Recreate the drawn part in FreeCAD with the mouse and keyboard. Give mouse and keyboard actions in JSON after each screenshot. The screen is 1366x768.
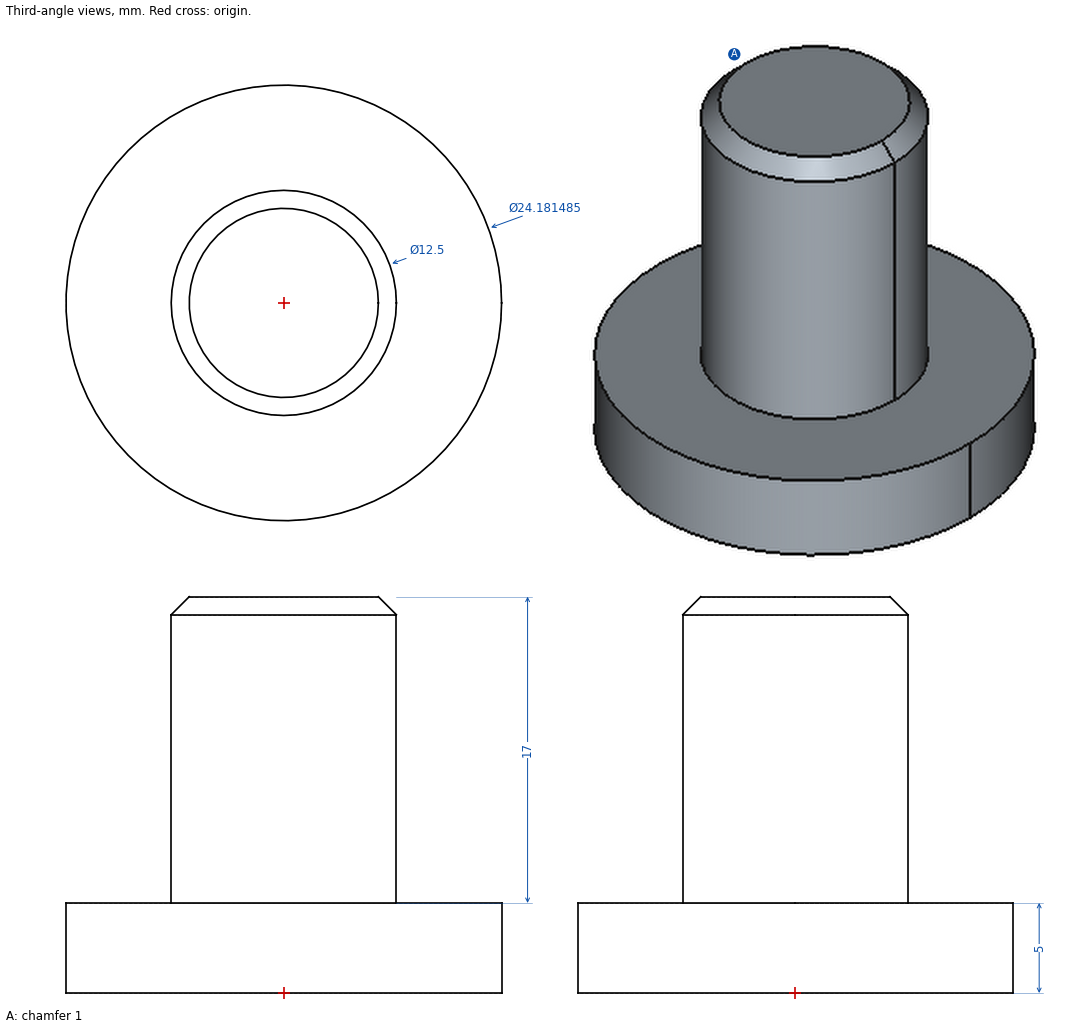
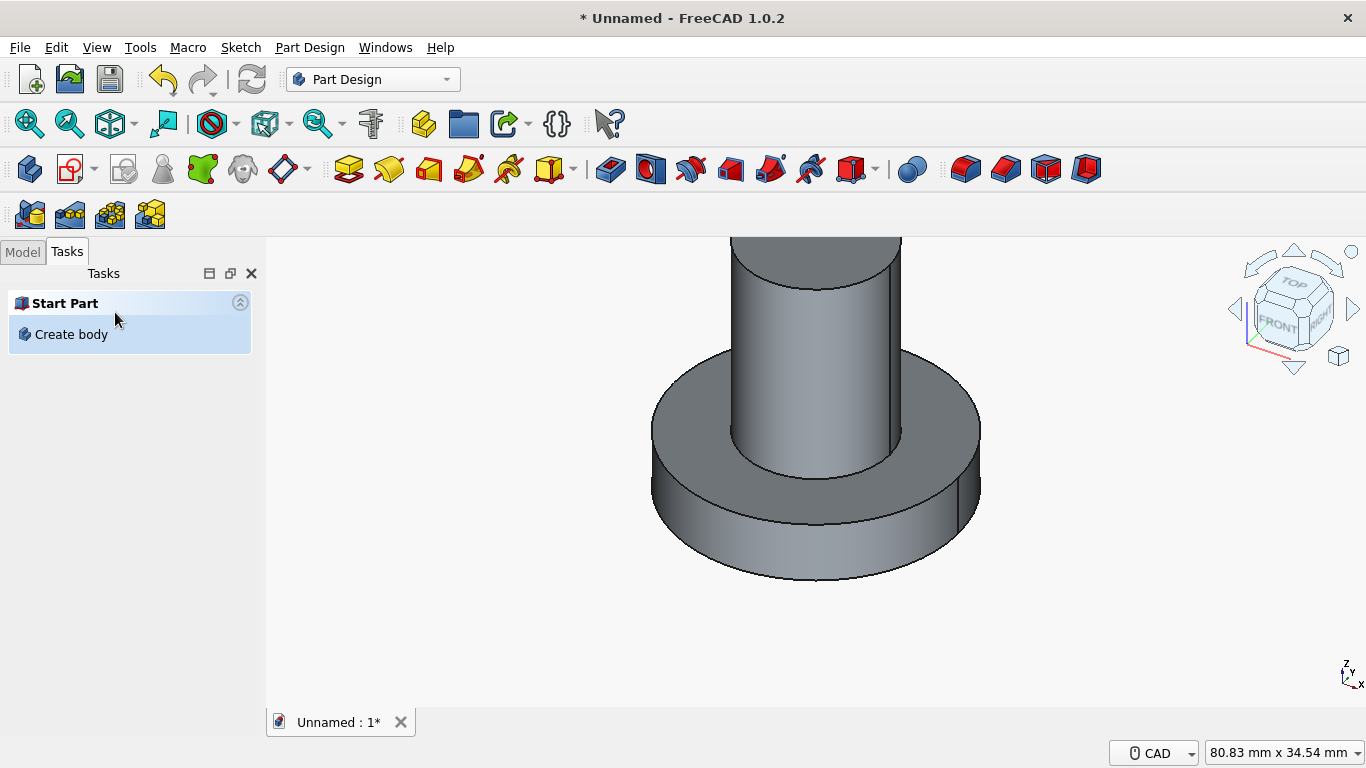
{"action": "left_click", "coordinate": [30, 124]}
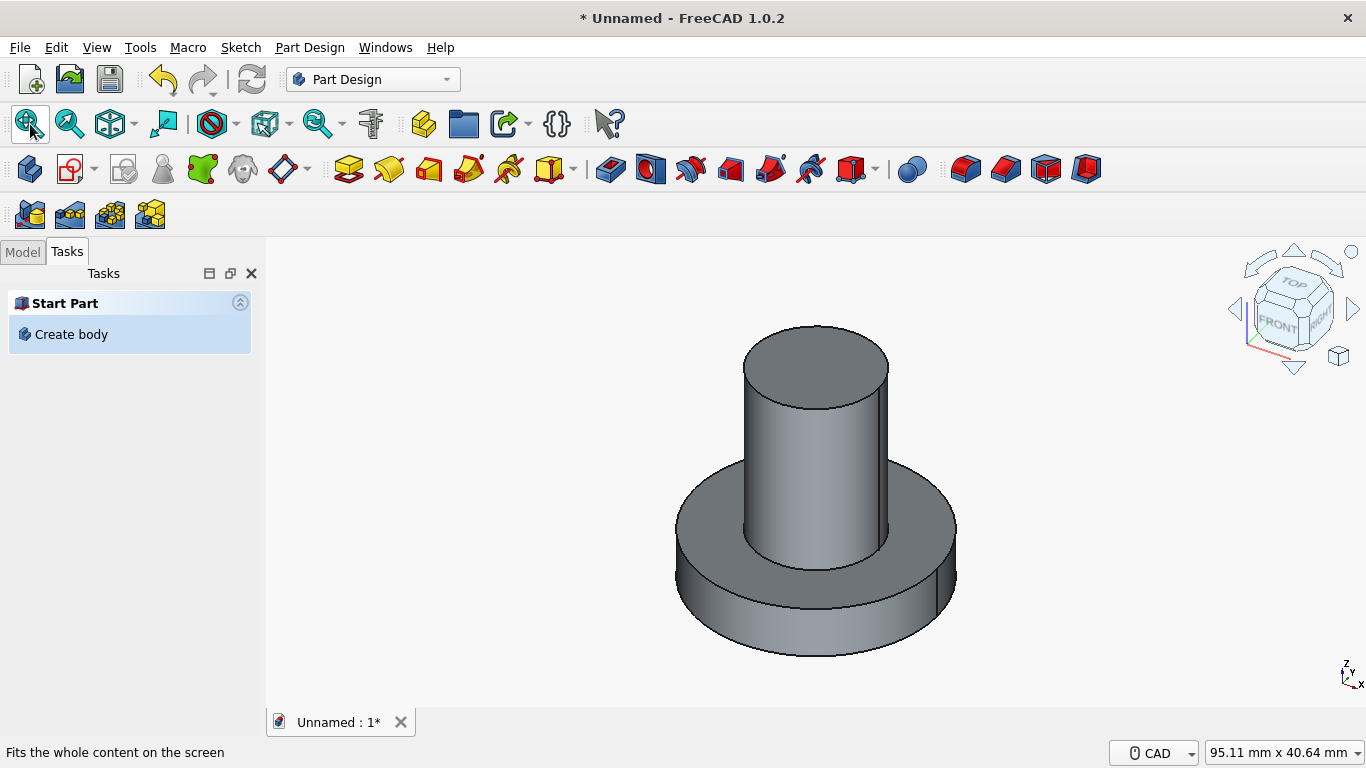
{"action": "left_click", "coordinate": [744, 371]}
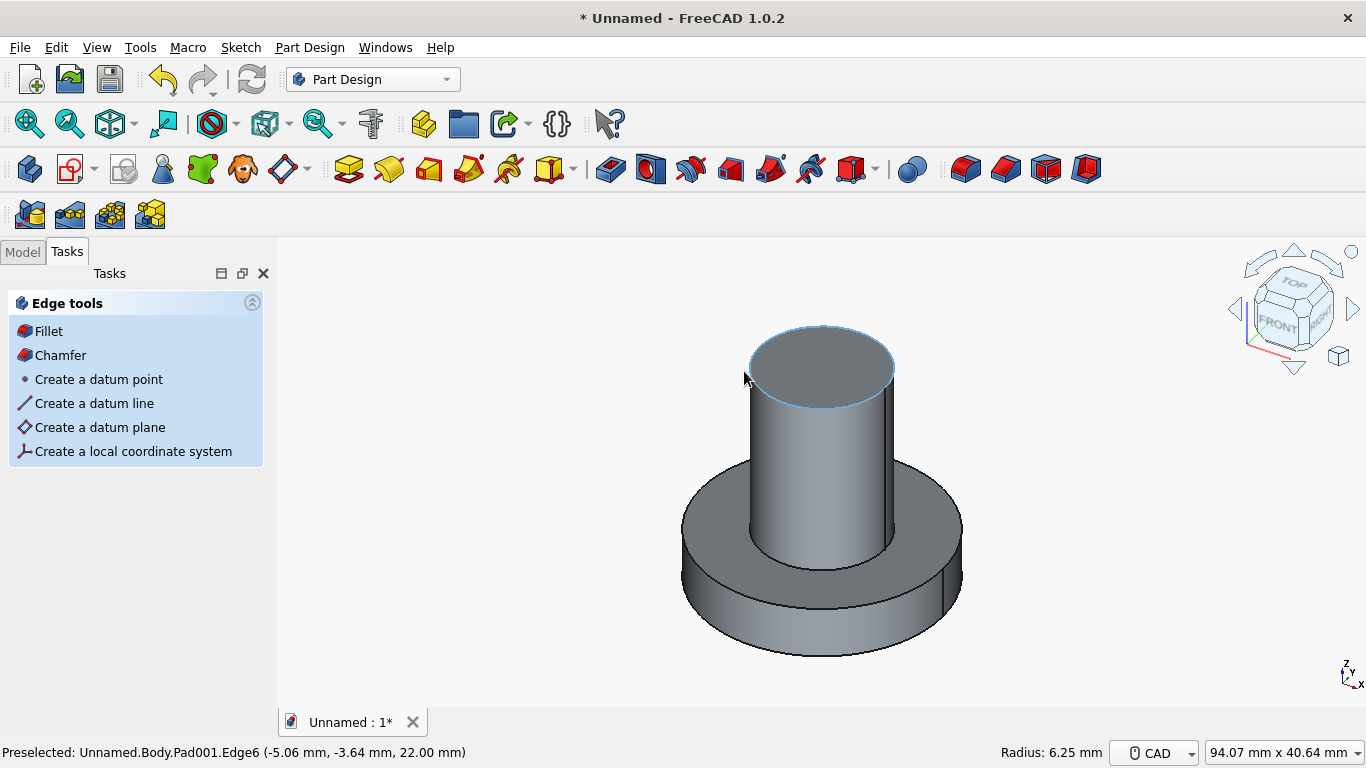
{"action": "left_click", "coordinate": [1006, 170]}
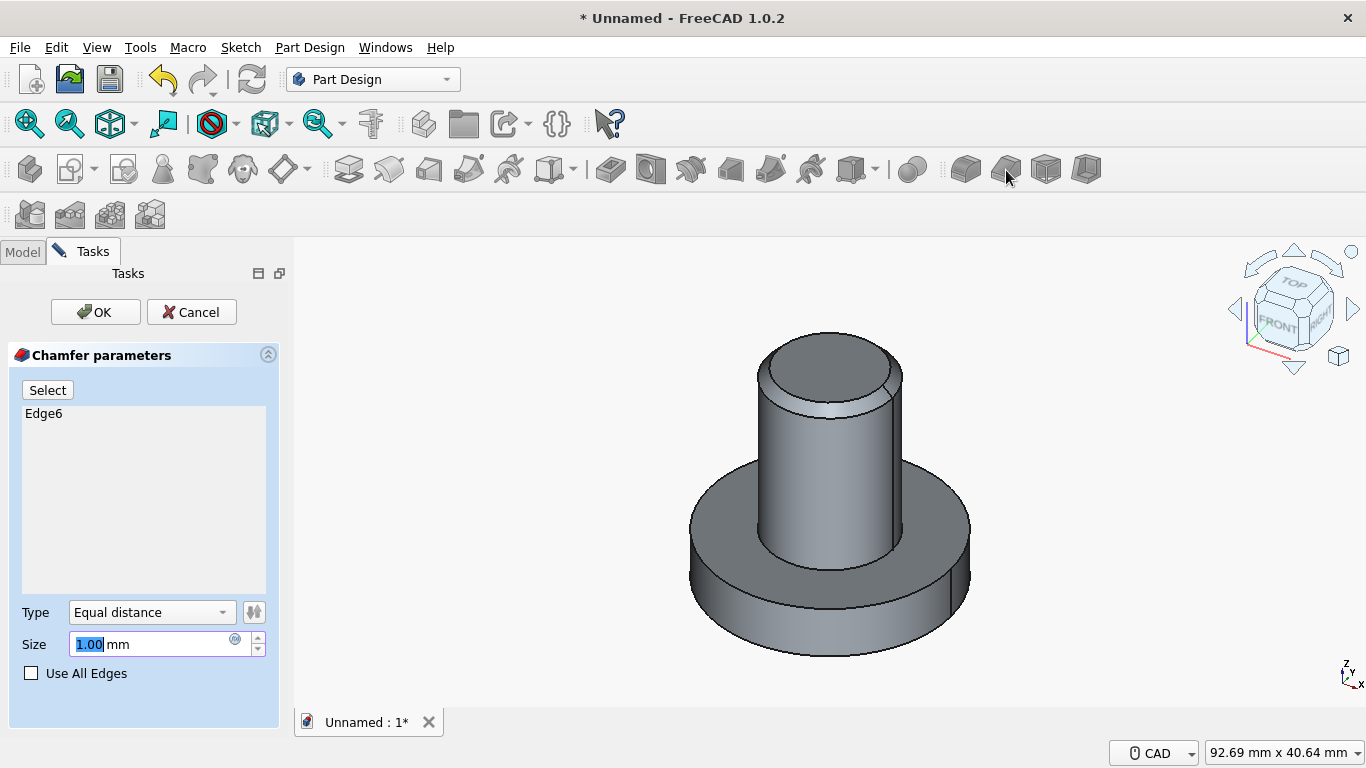
{"action": "type", "text": "1"}
{"action": "key", "text": "Tab"}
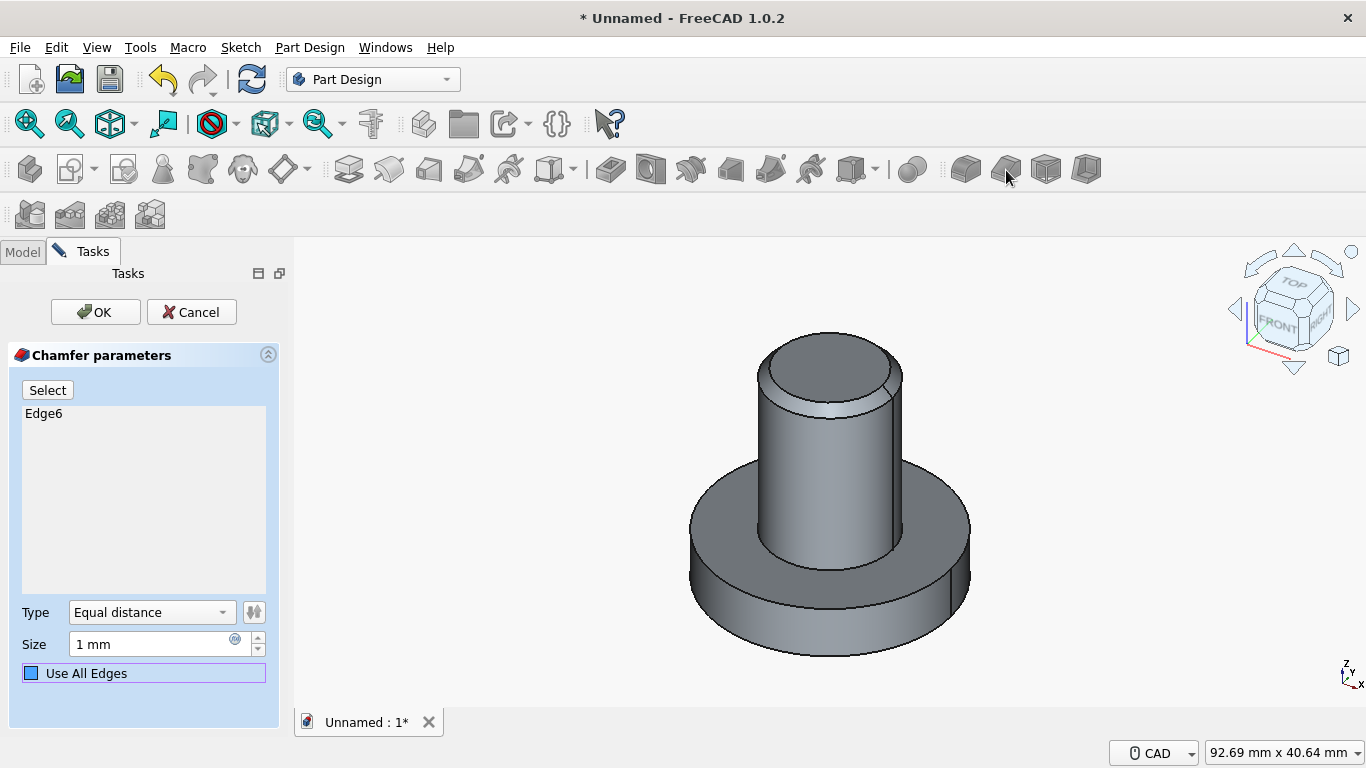
{"action": "left_click", "coordinate": [96, 312]}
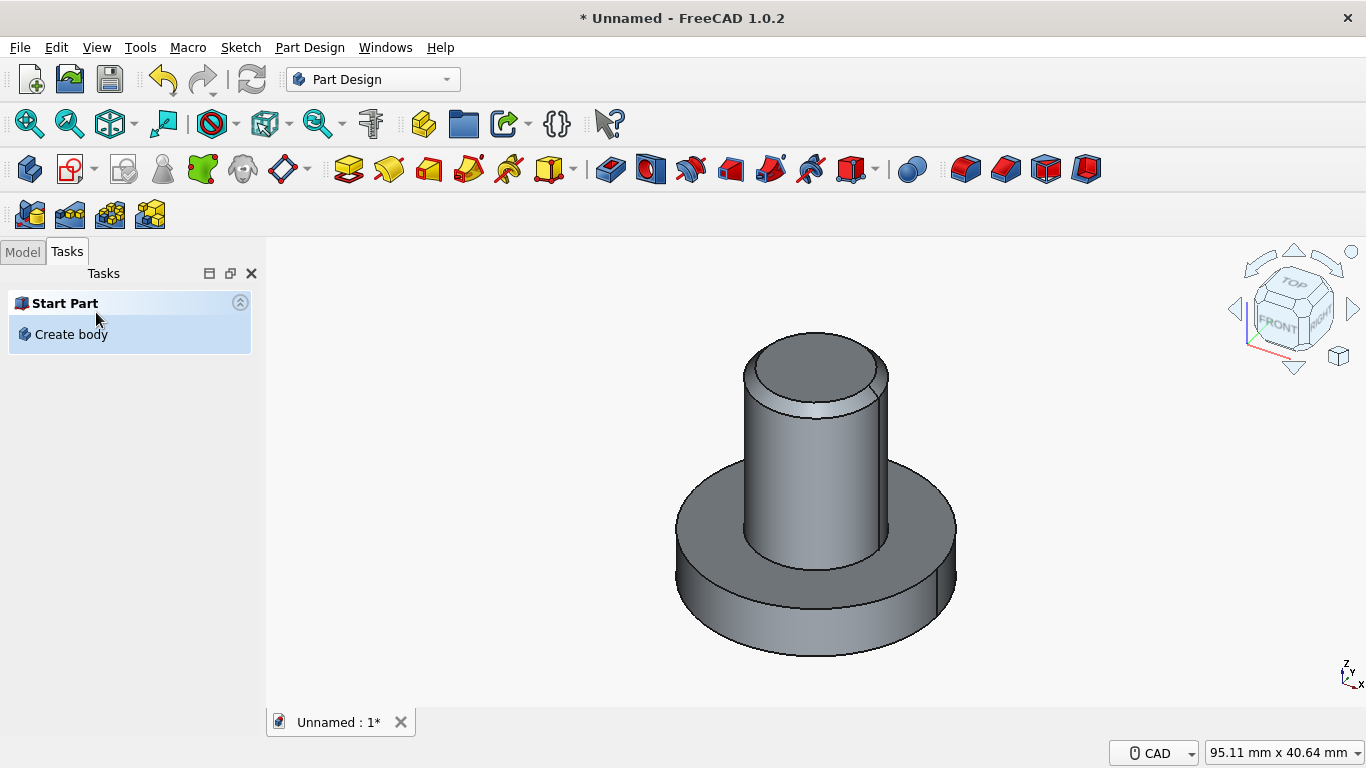
{"action": "key", "text": "0"}